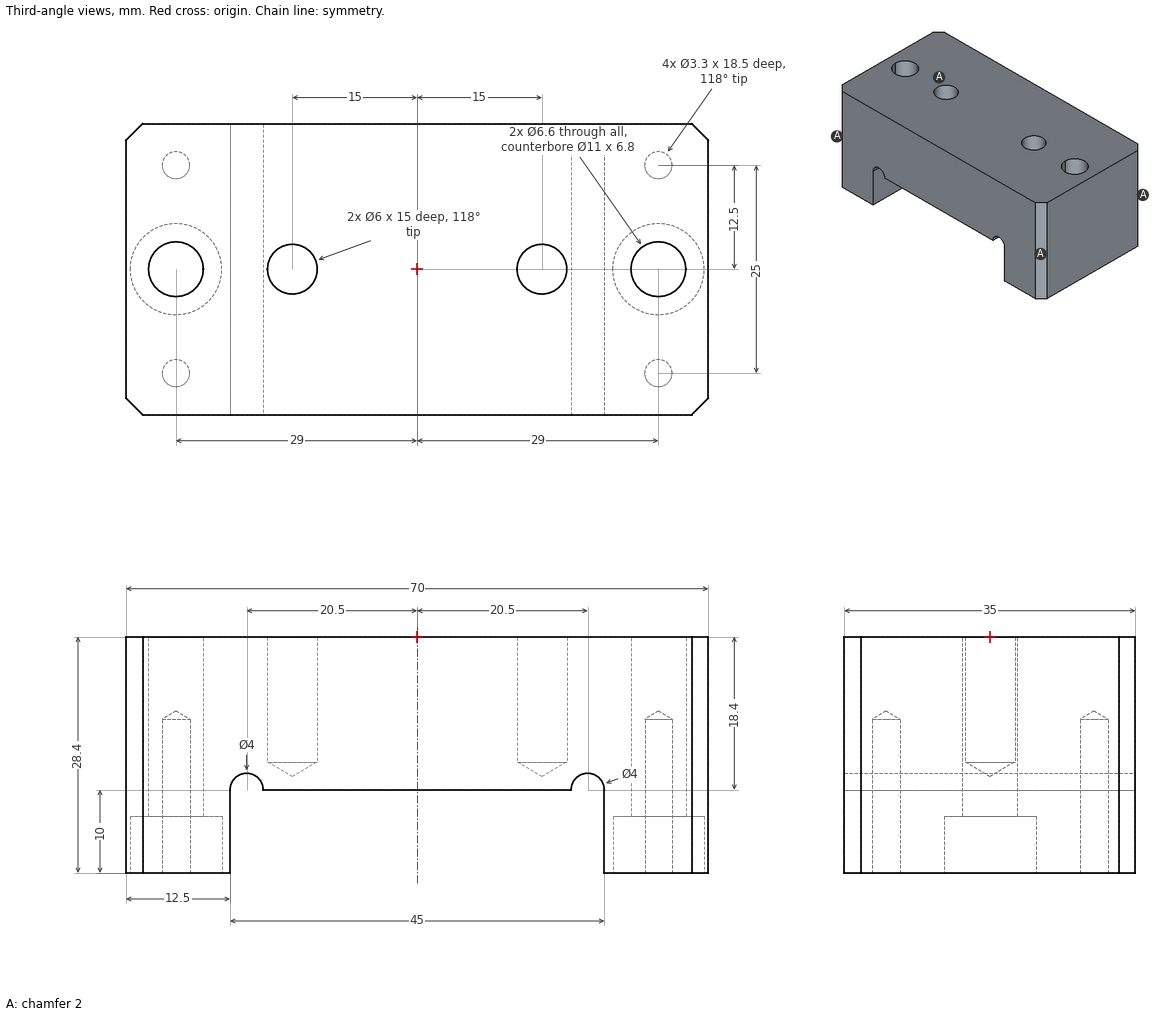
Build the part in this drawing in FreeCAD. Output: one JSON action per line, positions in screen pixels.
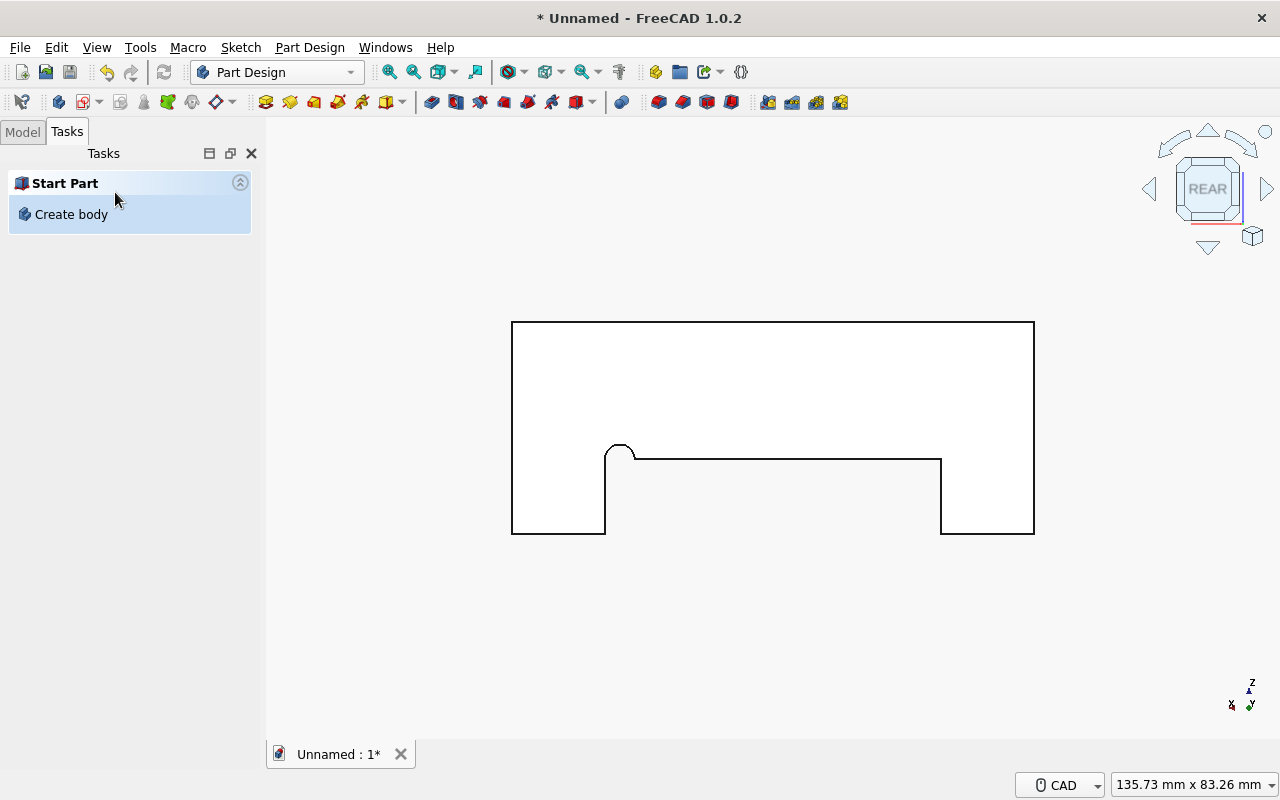
{"action": "left_click", "coordinate": [698, 397]}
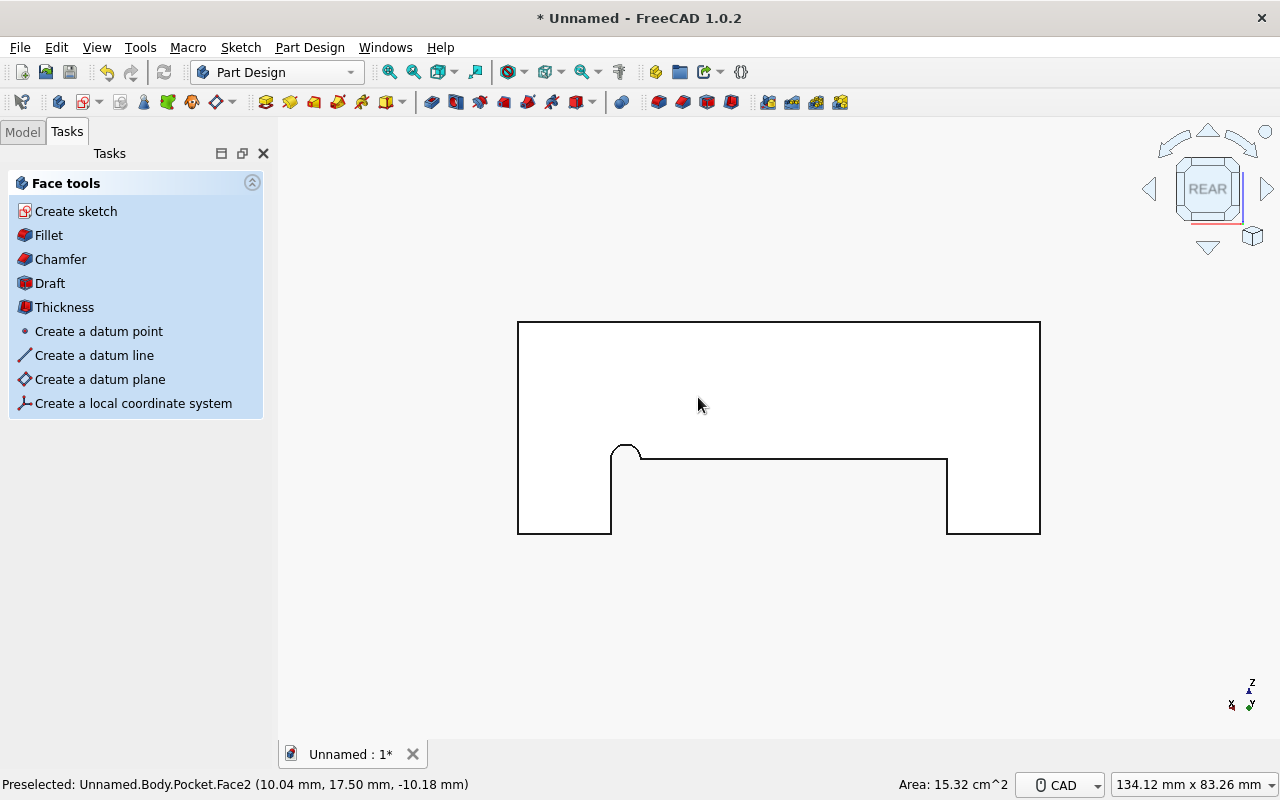
{"action": "left_click", "coordinate": [84, 102]}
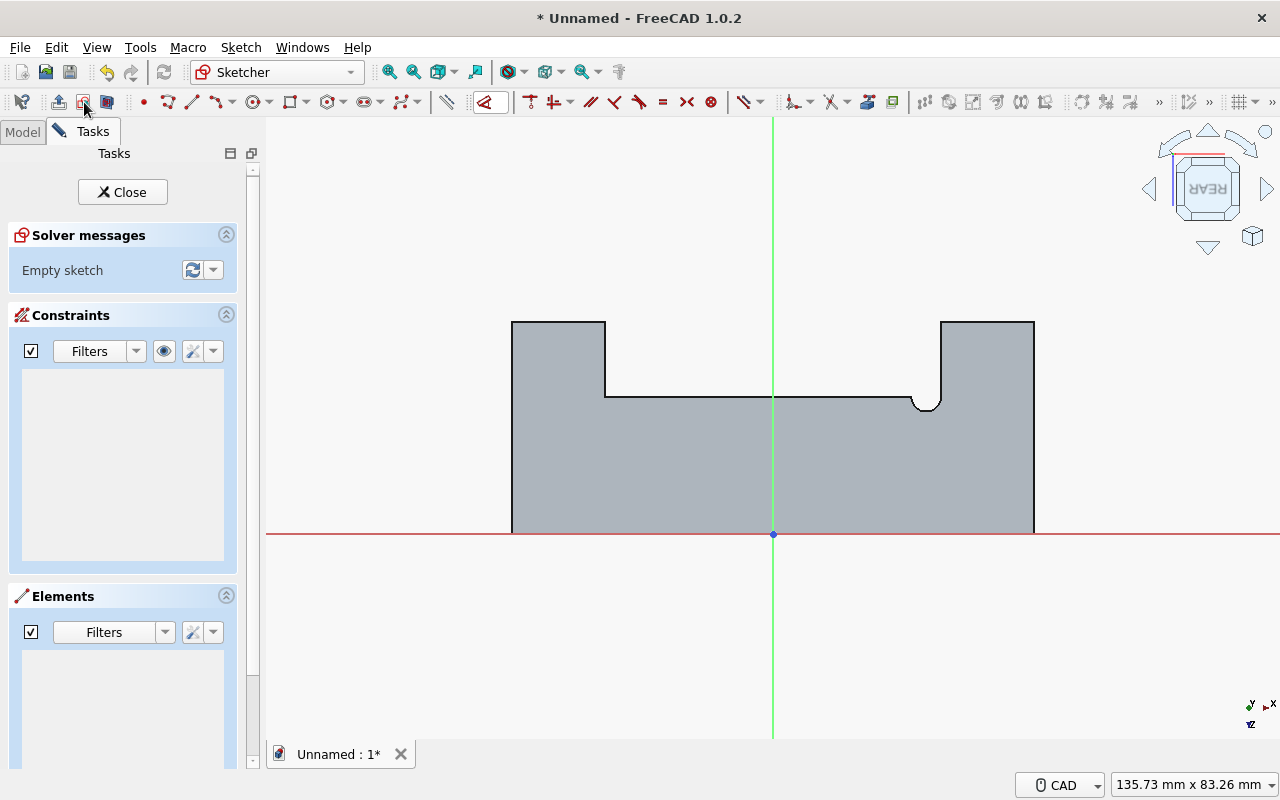
{"action": "scroll", "coordinate": [613, 394], "scroll_direction": "up", "scroll_amount": 13}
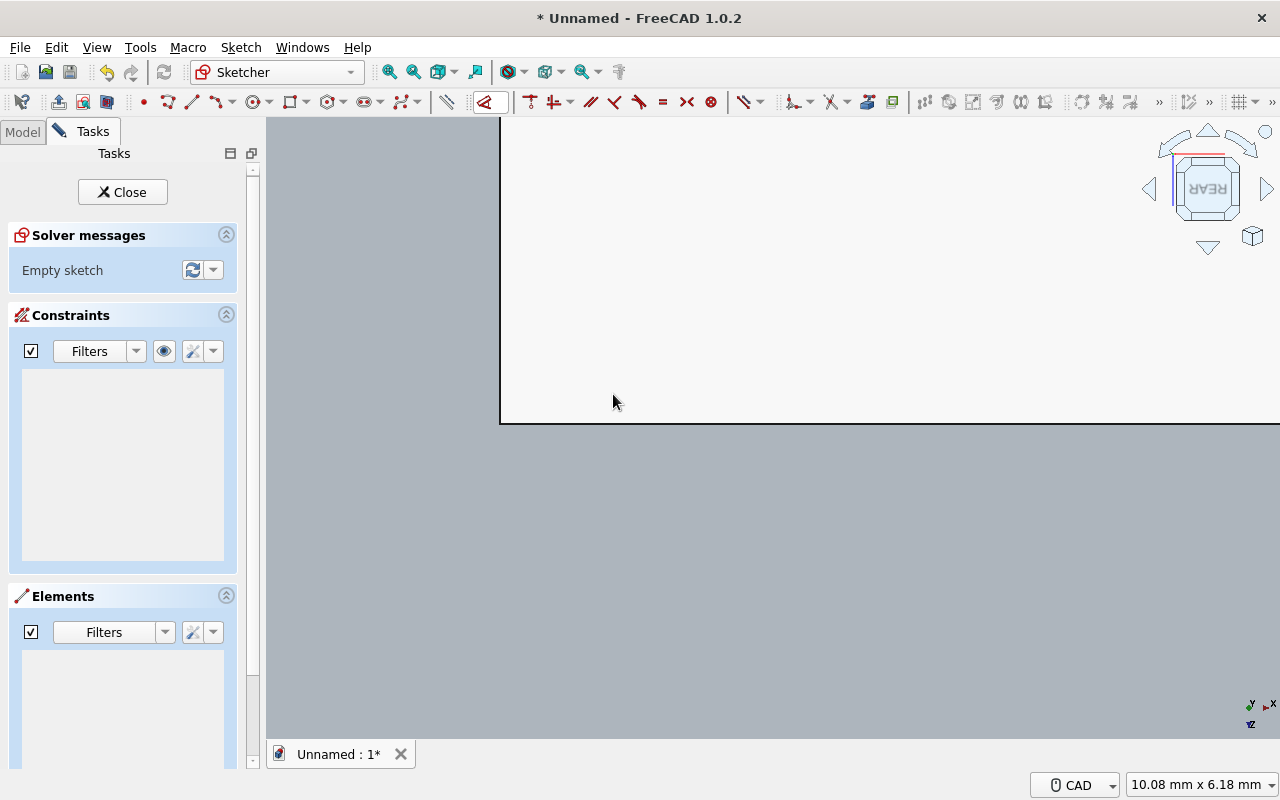
{"action": "left_click", "coordinate": [254, 102]}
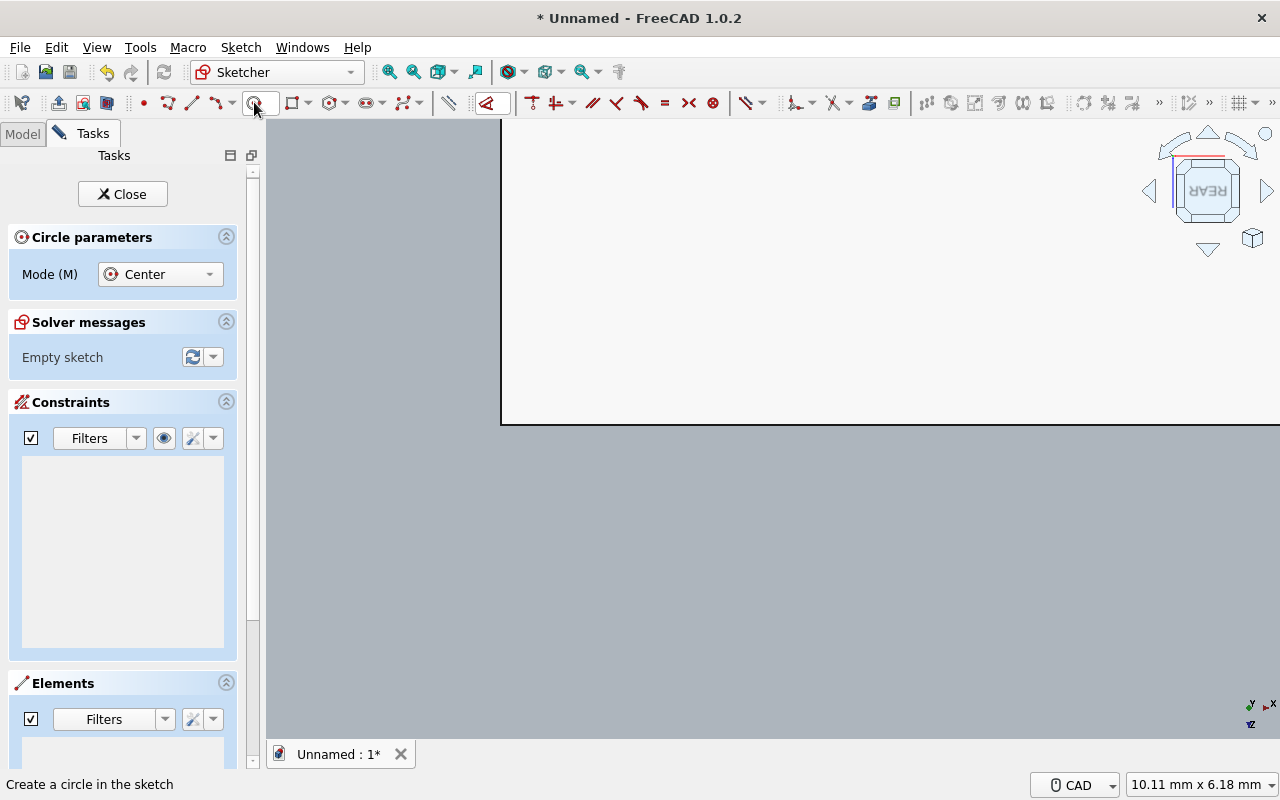
{"action": "left_click", "coordinate": [701, 425]}
{"action": "left_click", "coordinate": [843, 283]}
{"action": "key", "text": "Escape"}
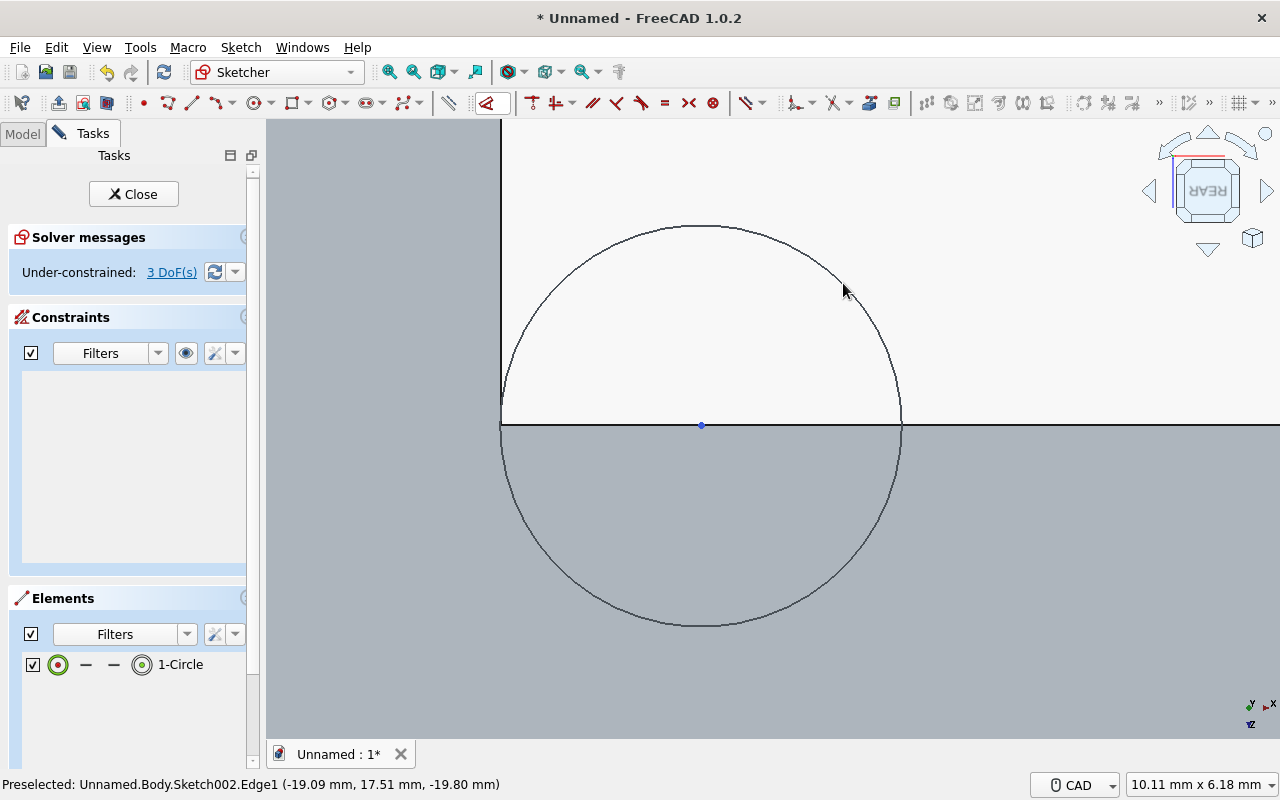
{"action": "key", "text": "d"}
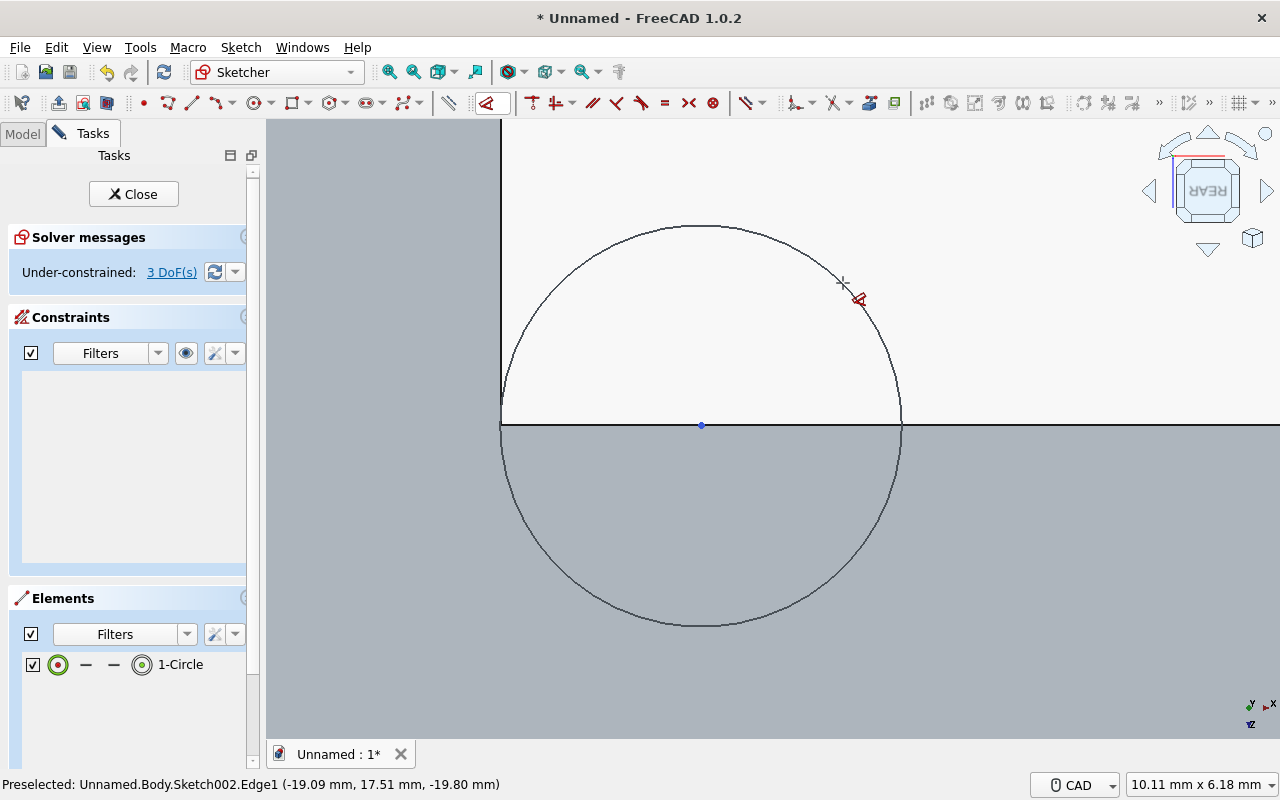
{"action": "left_click", "coordinate": [843, 284]}
{"action": "left_click", "coordinate": [866, 261]}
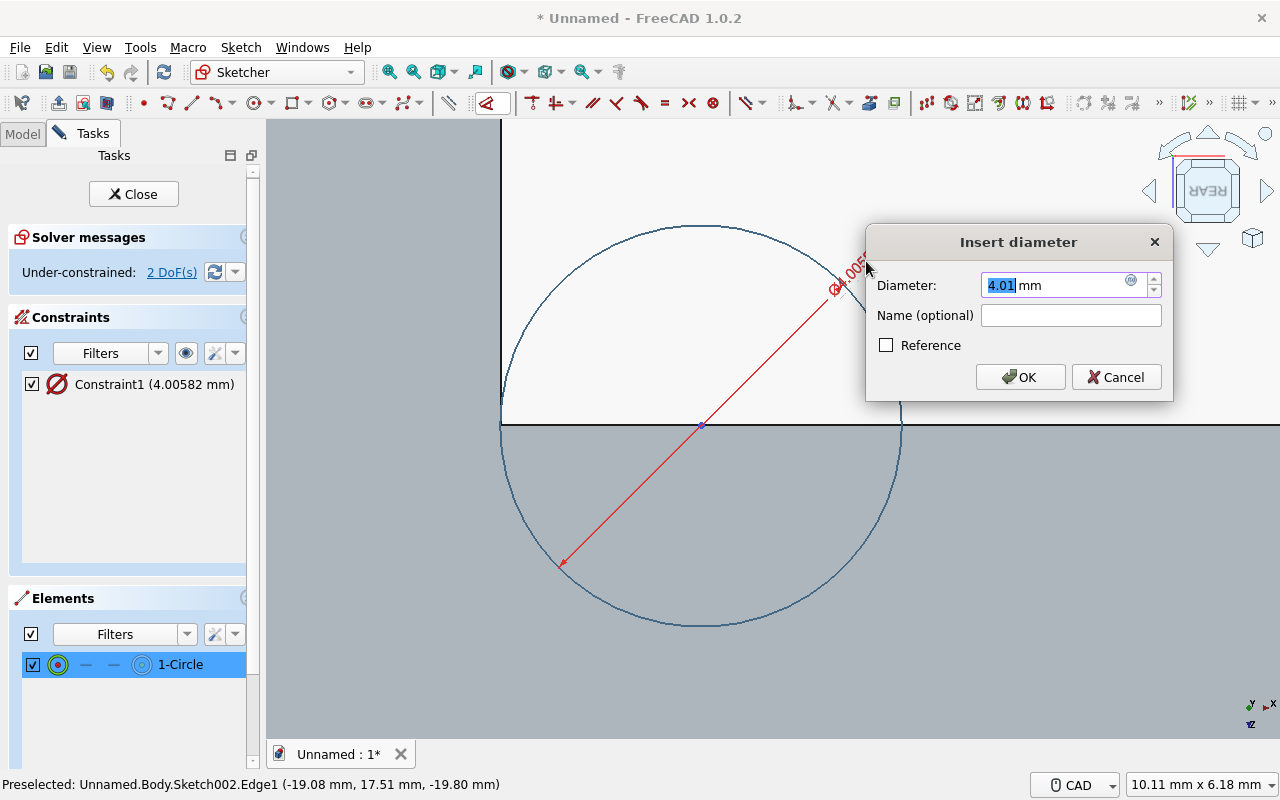
{"action": "type", "text": "4"}
{"action": "key", "text": "Return"}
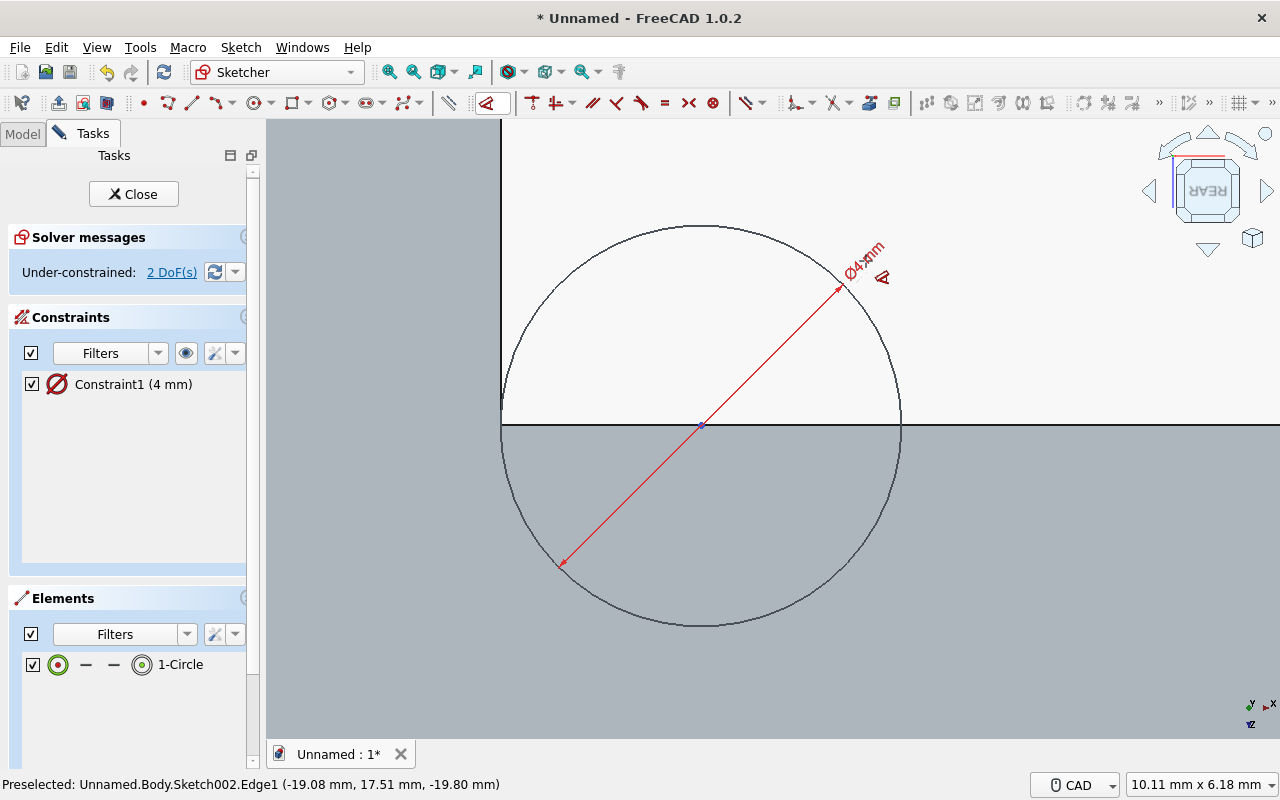
{"action": "left_click", "coordinate": [701, 426]}
{"action": "left_click", "coordinate": [813, 392]}